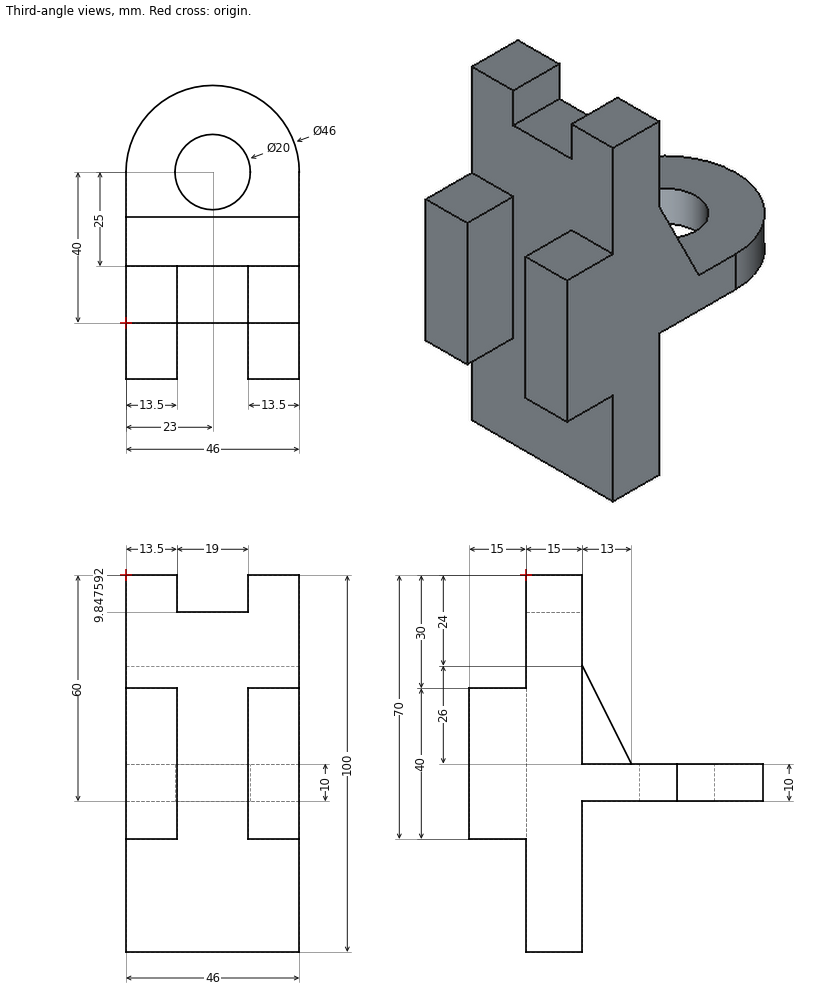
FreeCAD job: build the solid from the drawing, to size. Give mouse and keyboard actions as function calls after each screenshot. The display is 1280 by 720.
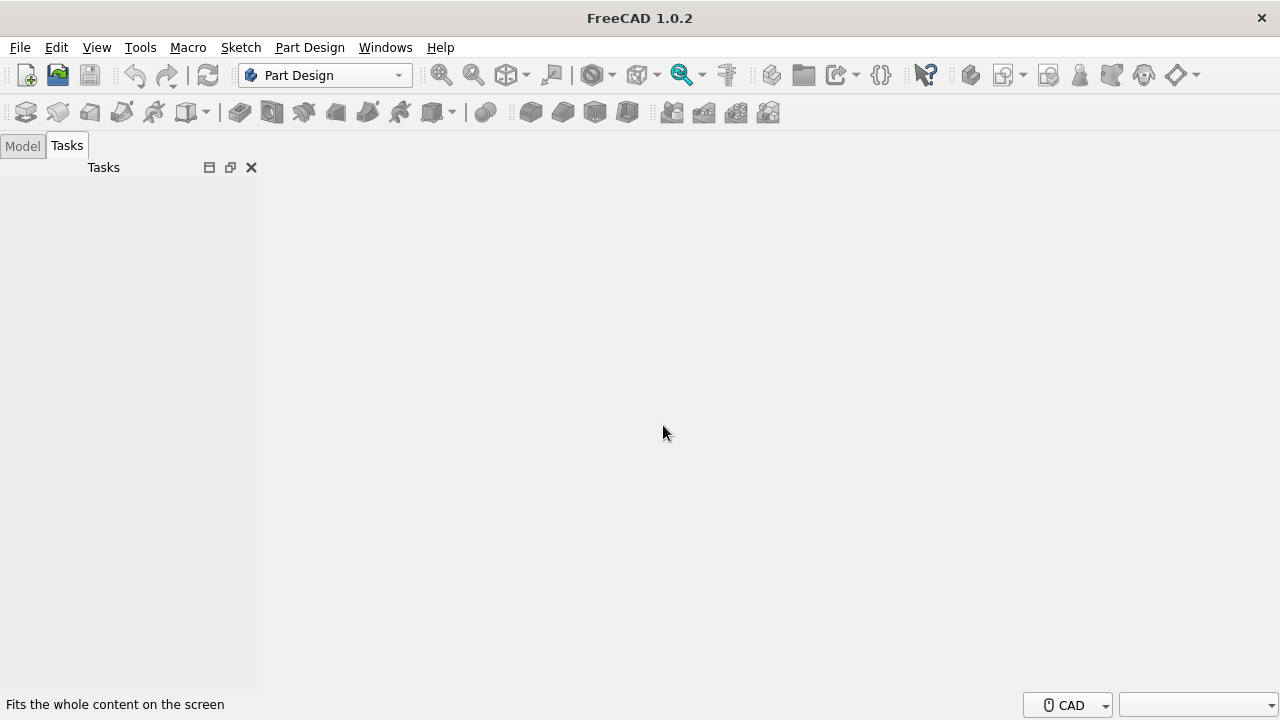
click(26, 76)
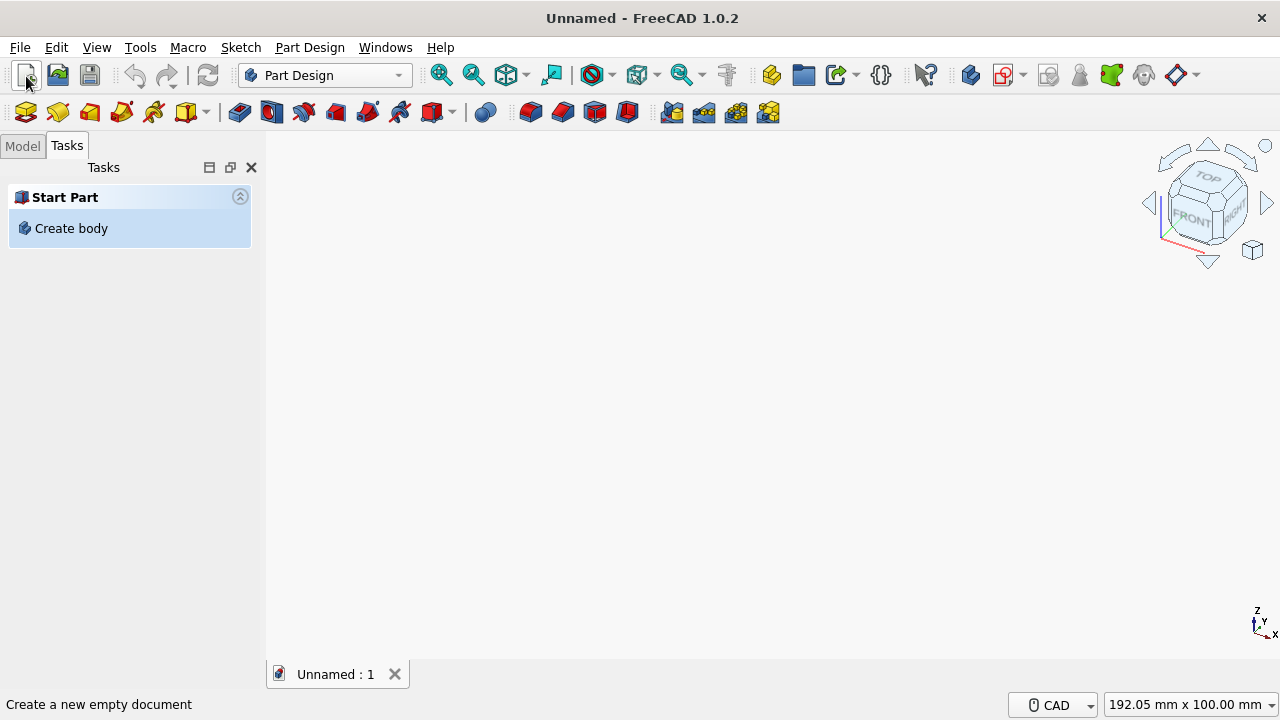
click(1004, 76)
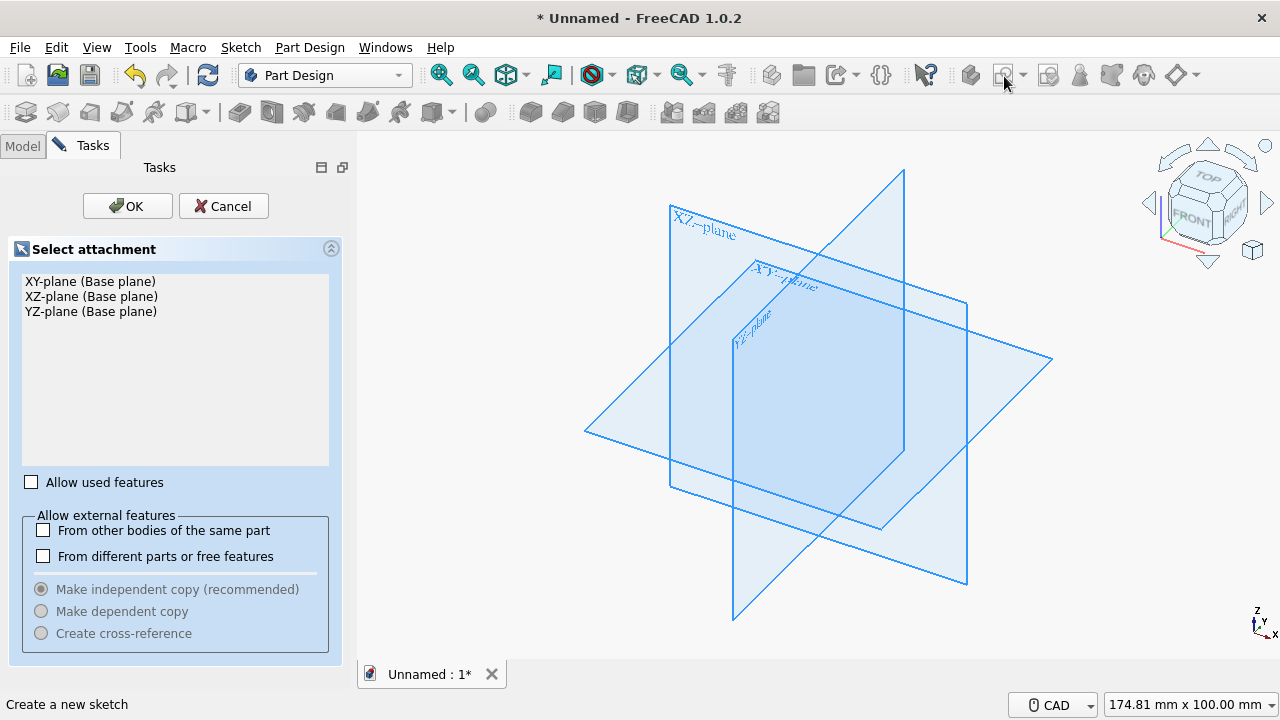
click(82, 296)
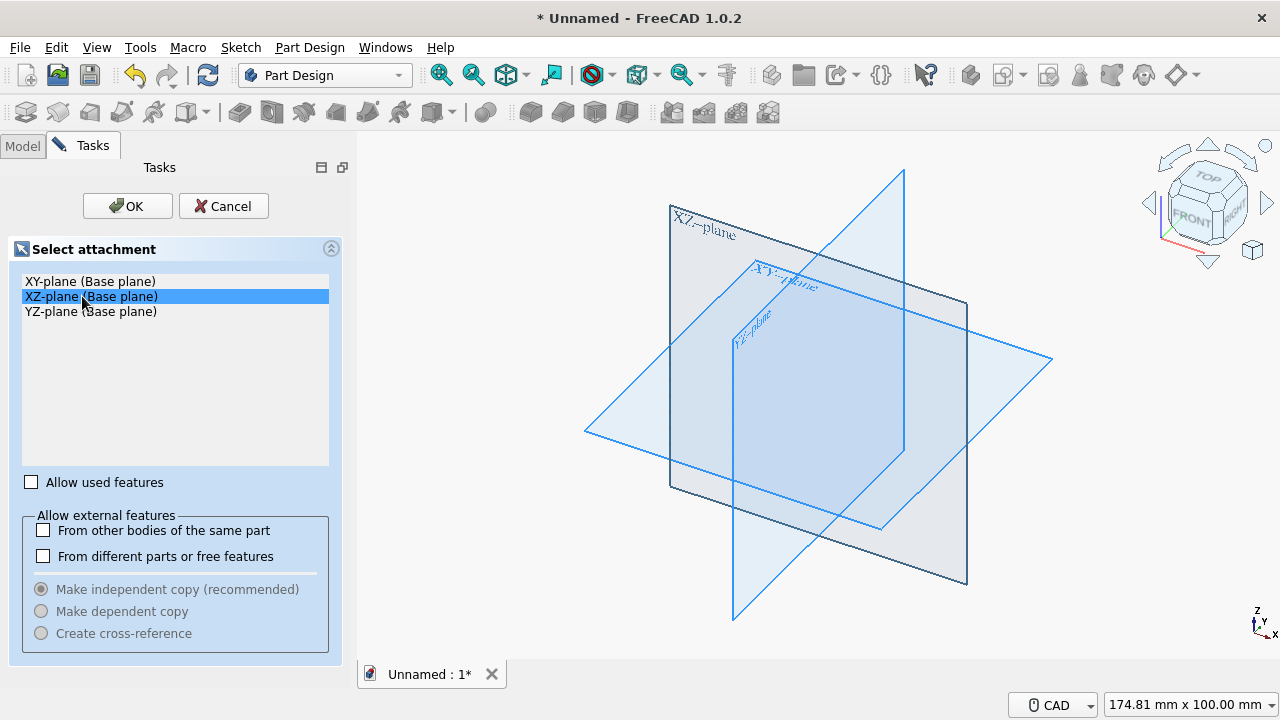
click(128, 206)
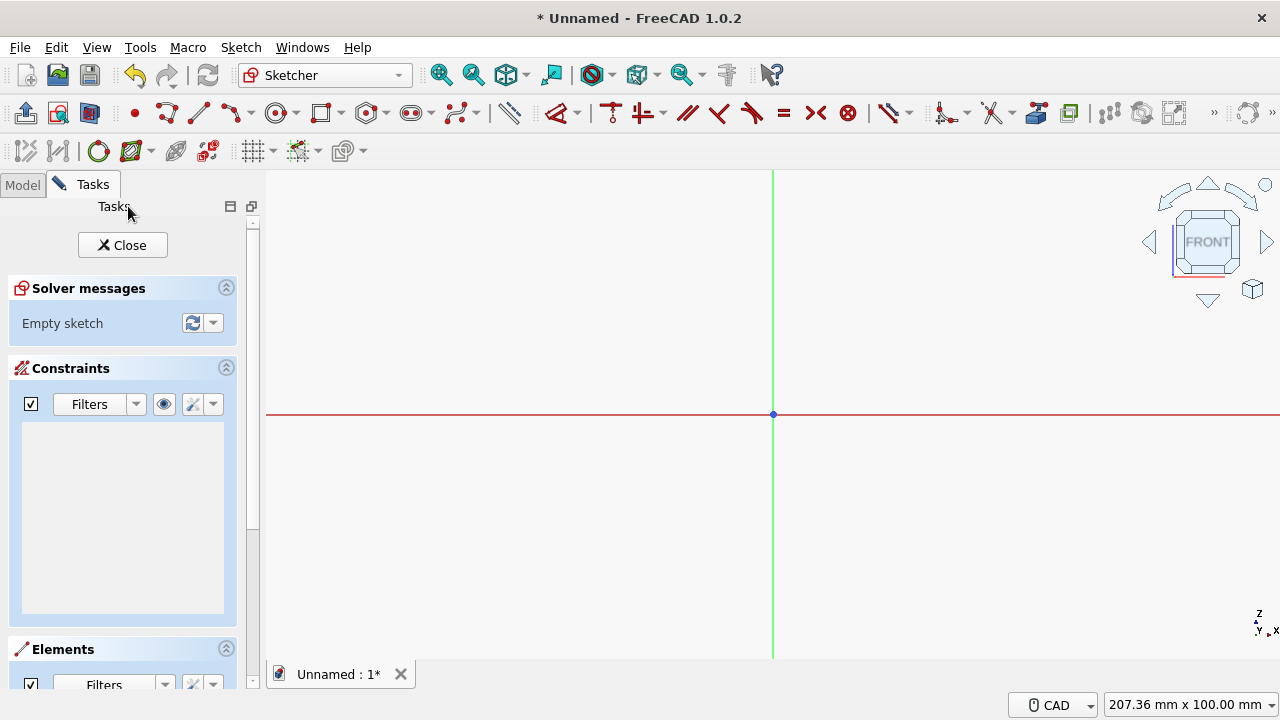
scroll(484, 198, down, 3)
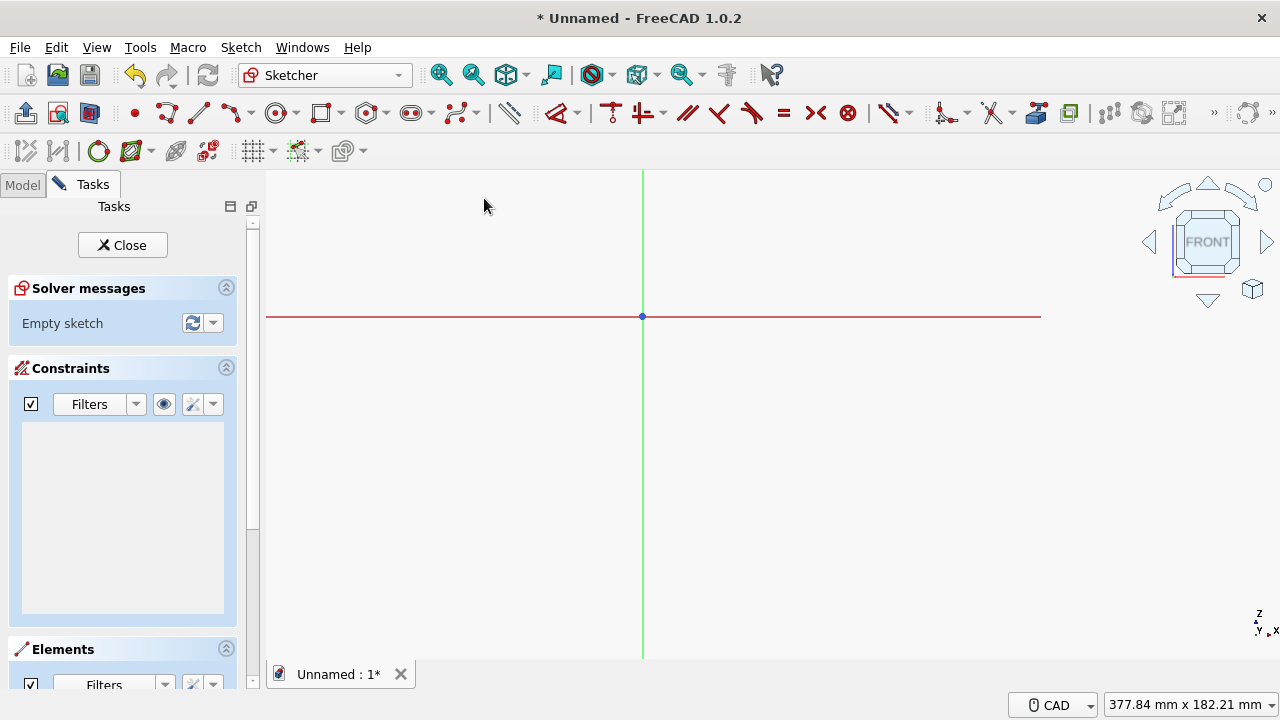
key(g)
key(m)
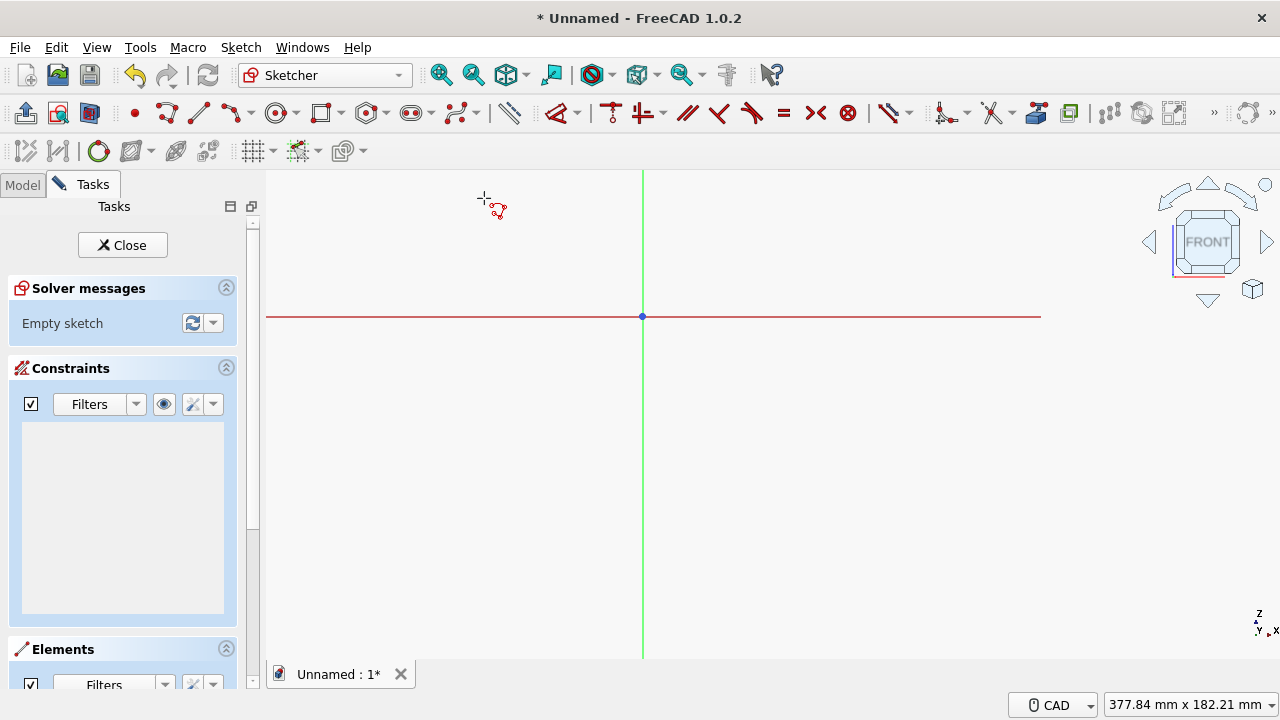
click(643, 317)
click(679, 326)
click(679, 343)
click(730, 343)
click(730, 317)
click(766, 326)
click(766, 585)
click(652, 585)
click(643, 317)
key(Escape)
key(Escape)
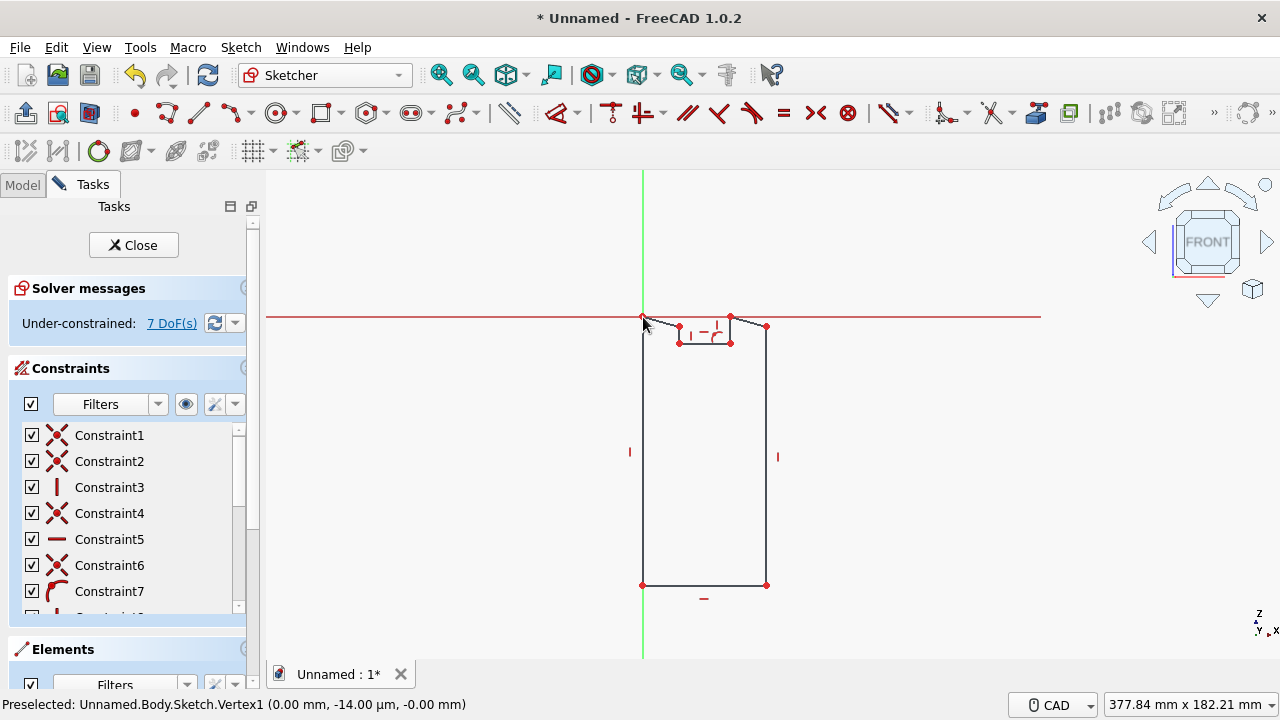
scroll(654, 320, up, 2)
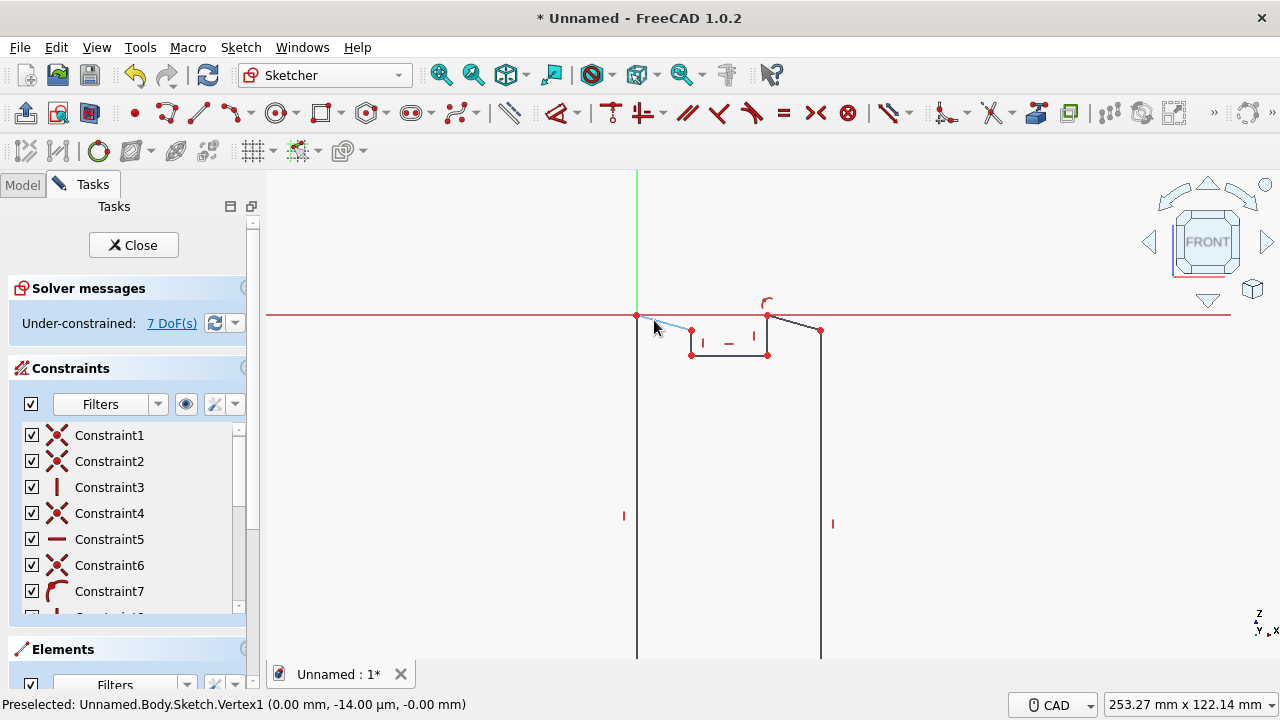
click(653, 320)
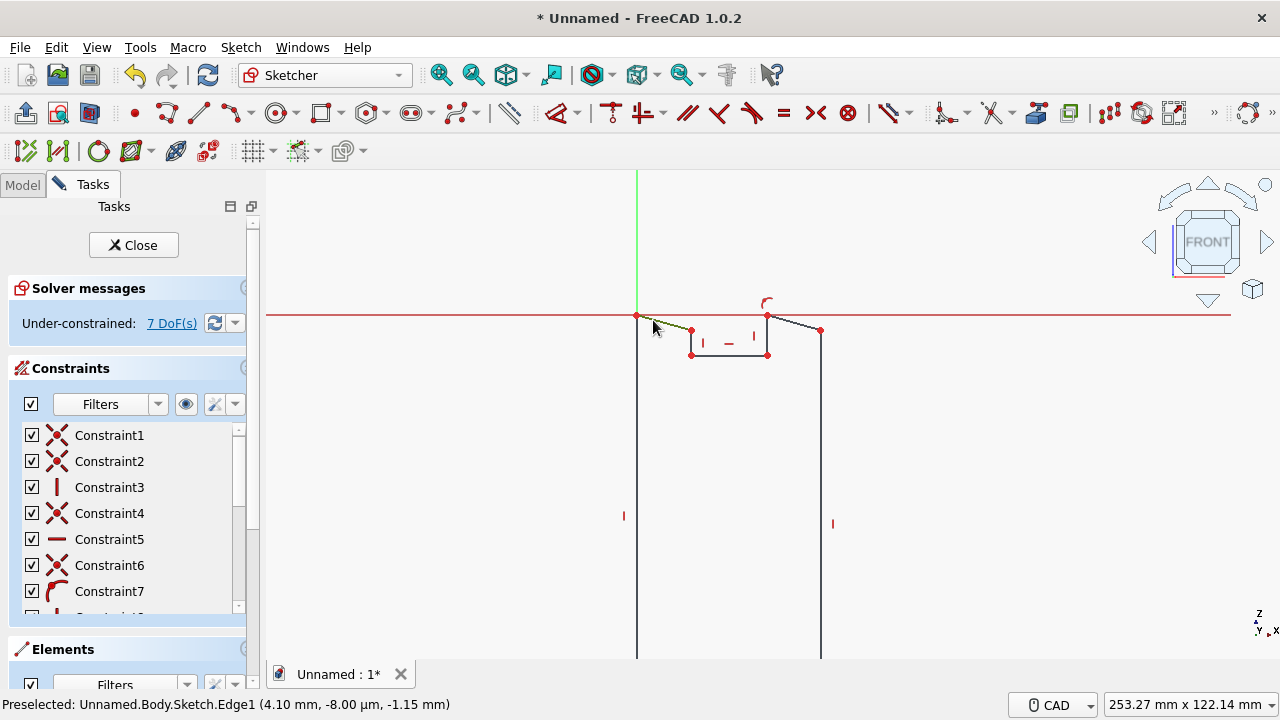
key(h)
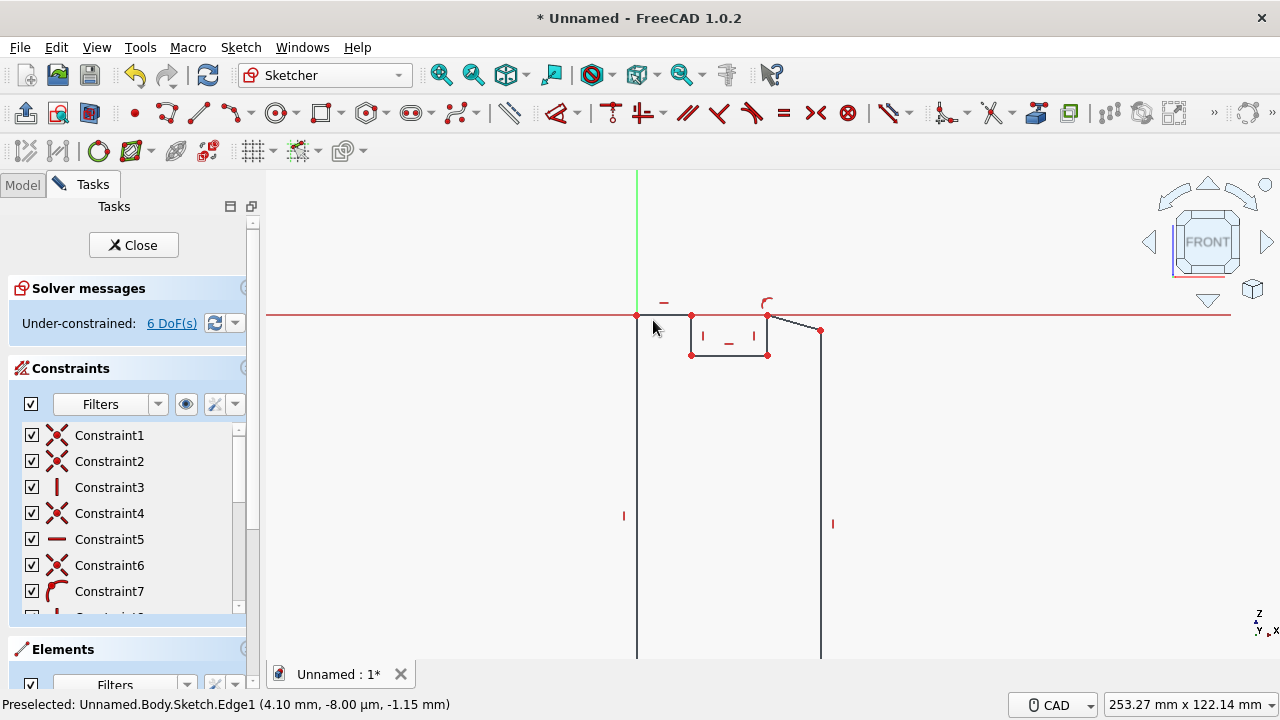
scroll(805, 326, up, 2)